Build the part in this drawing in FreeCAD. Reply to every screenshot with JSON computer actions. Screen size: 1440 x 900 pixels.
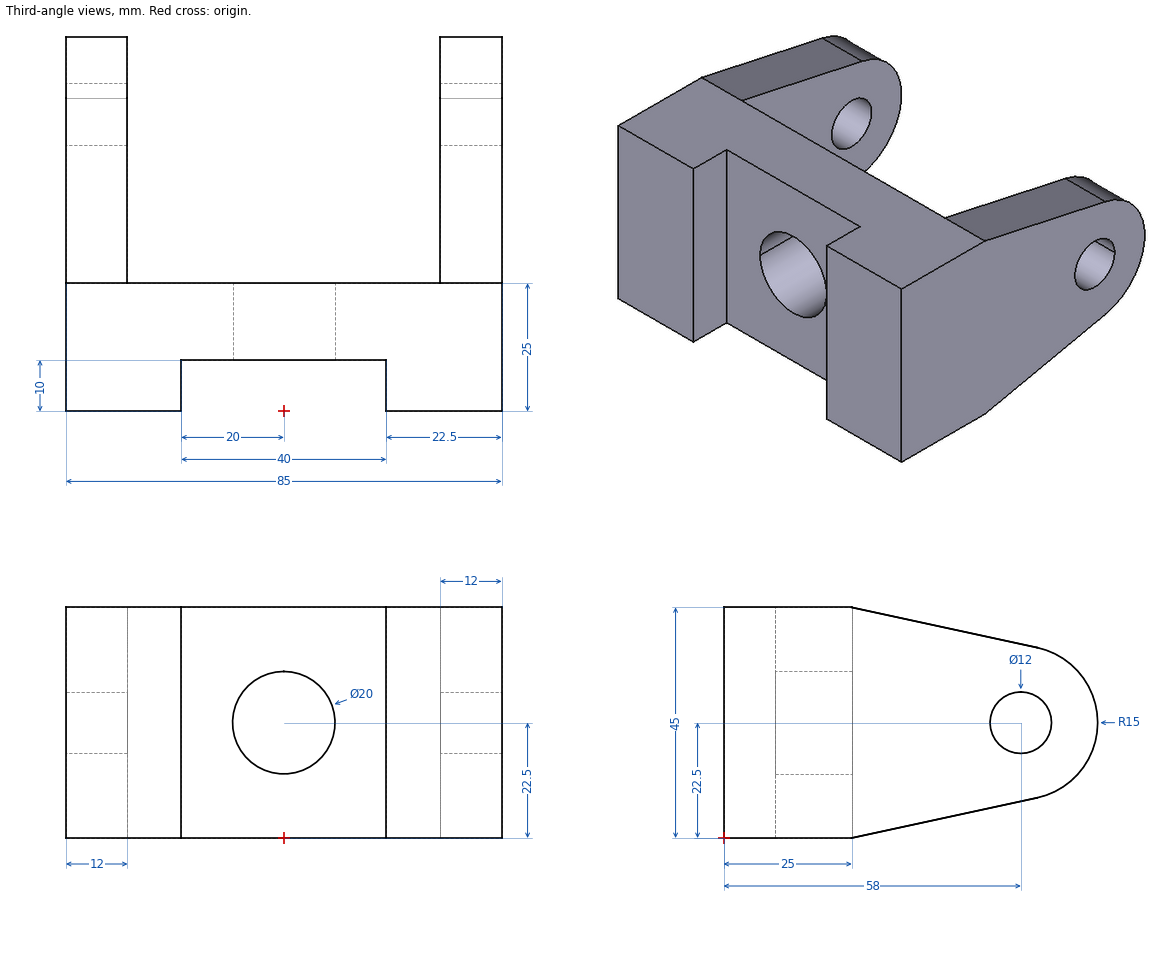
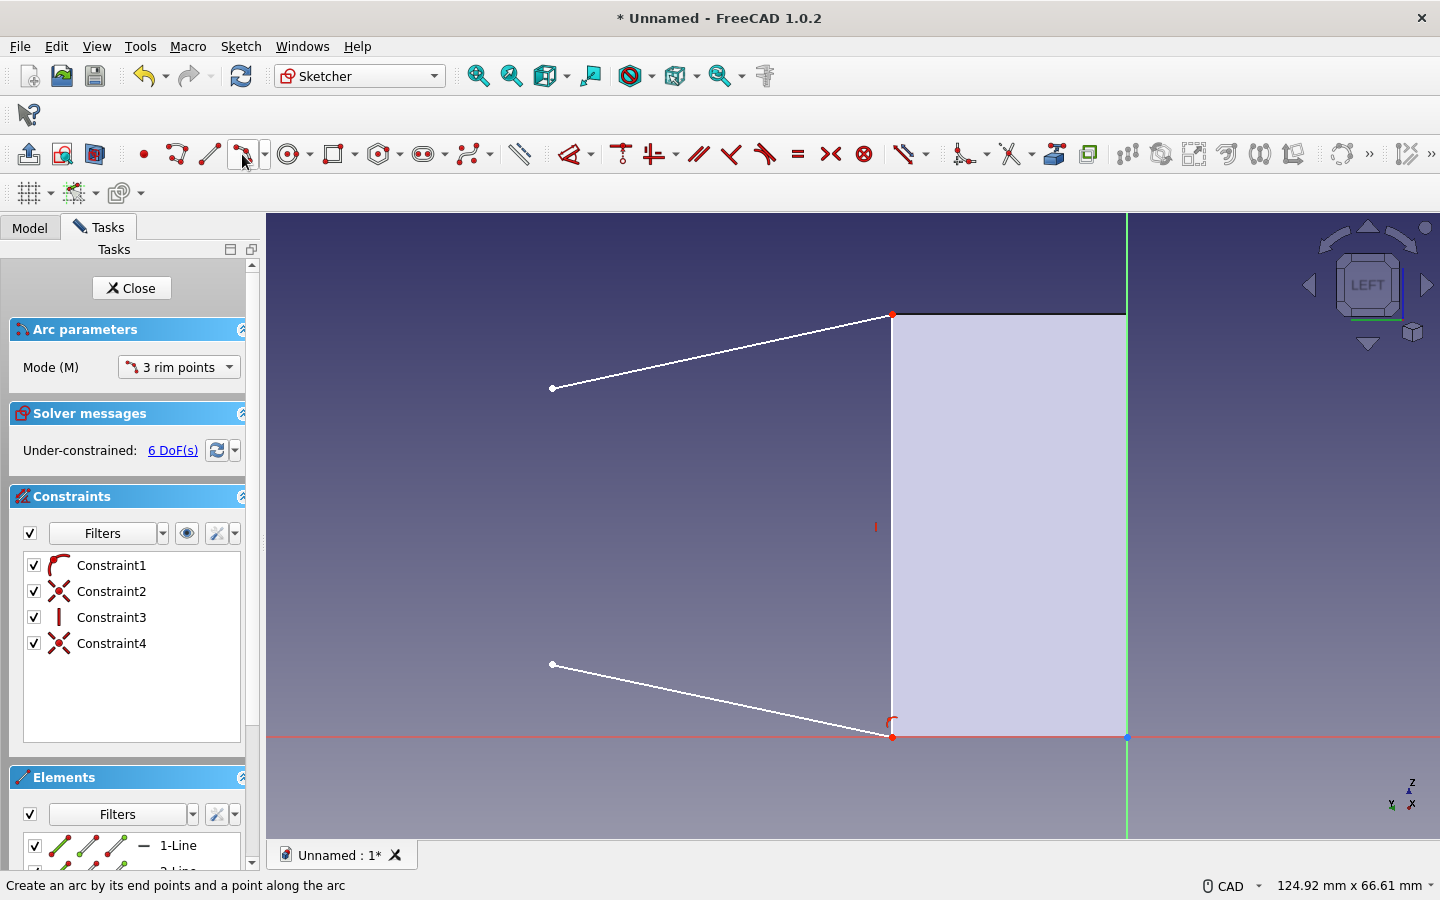
{"action": "left_click", "coordinate": [552, 389]}
{"action": "left_click", "coordinate": [552, 665]}
{"action": "left_click", "coordinate": [441, 526]}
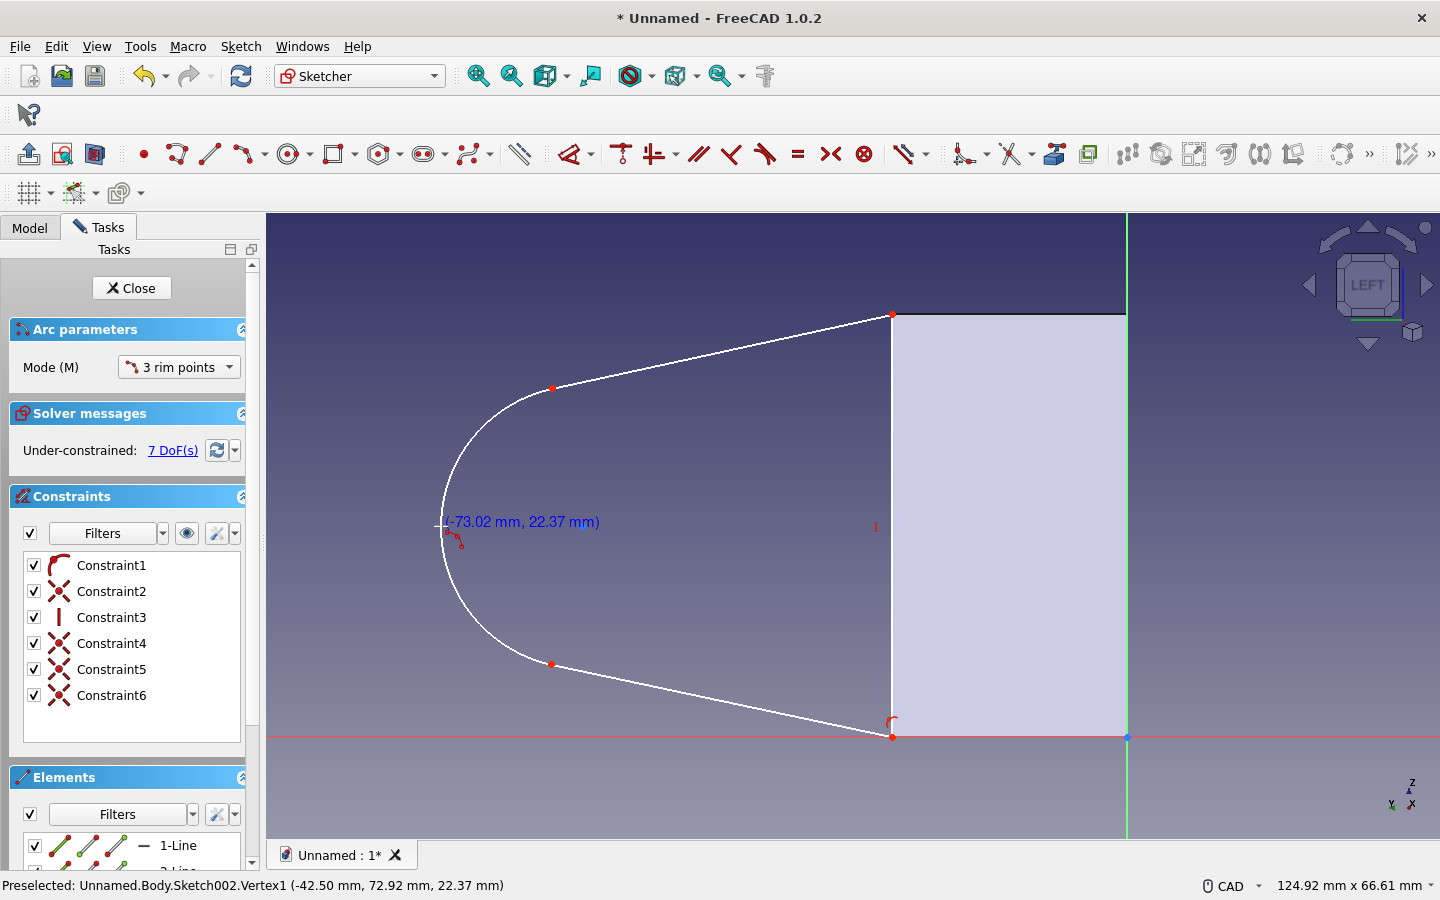
{"action": "left_click", "coordinate": [288, 154]}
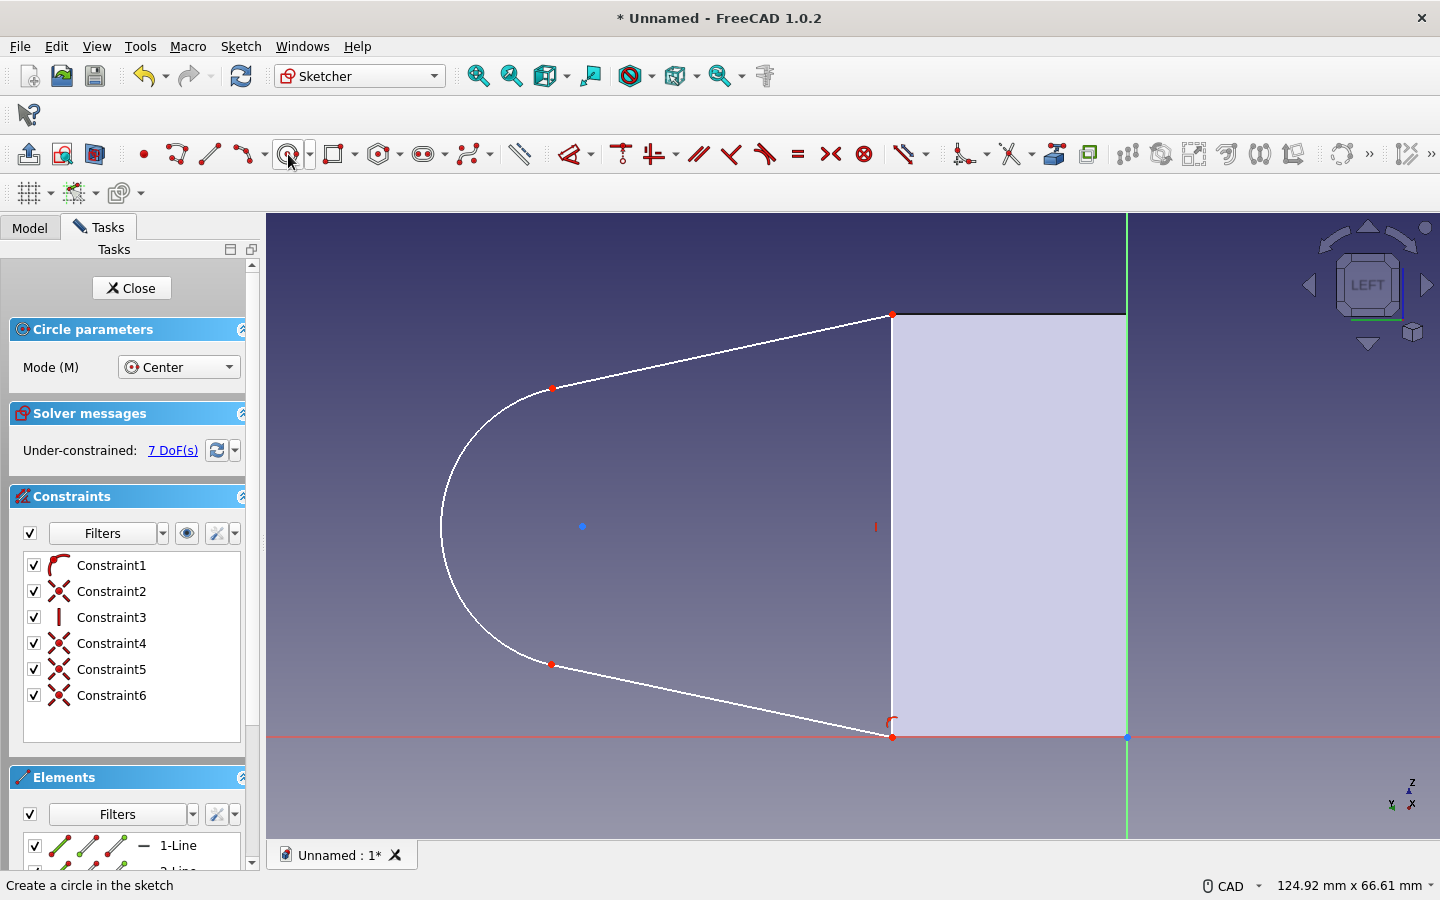
{"action": "left_click", "coordinate": [582, 526]}
{"action": "mouse_move", "coordinate": [622, 486]}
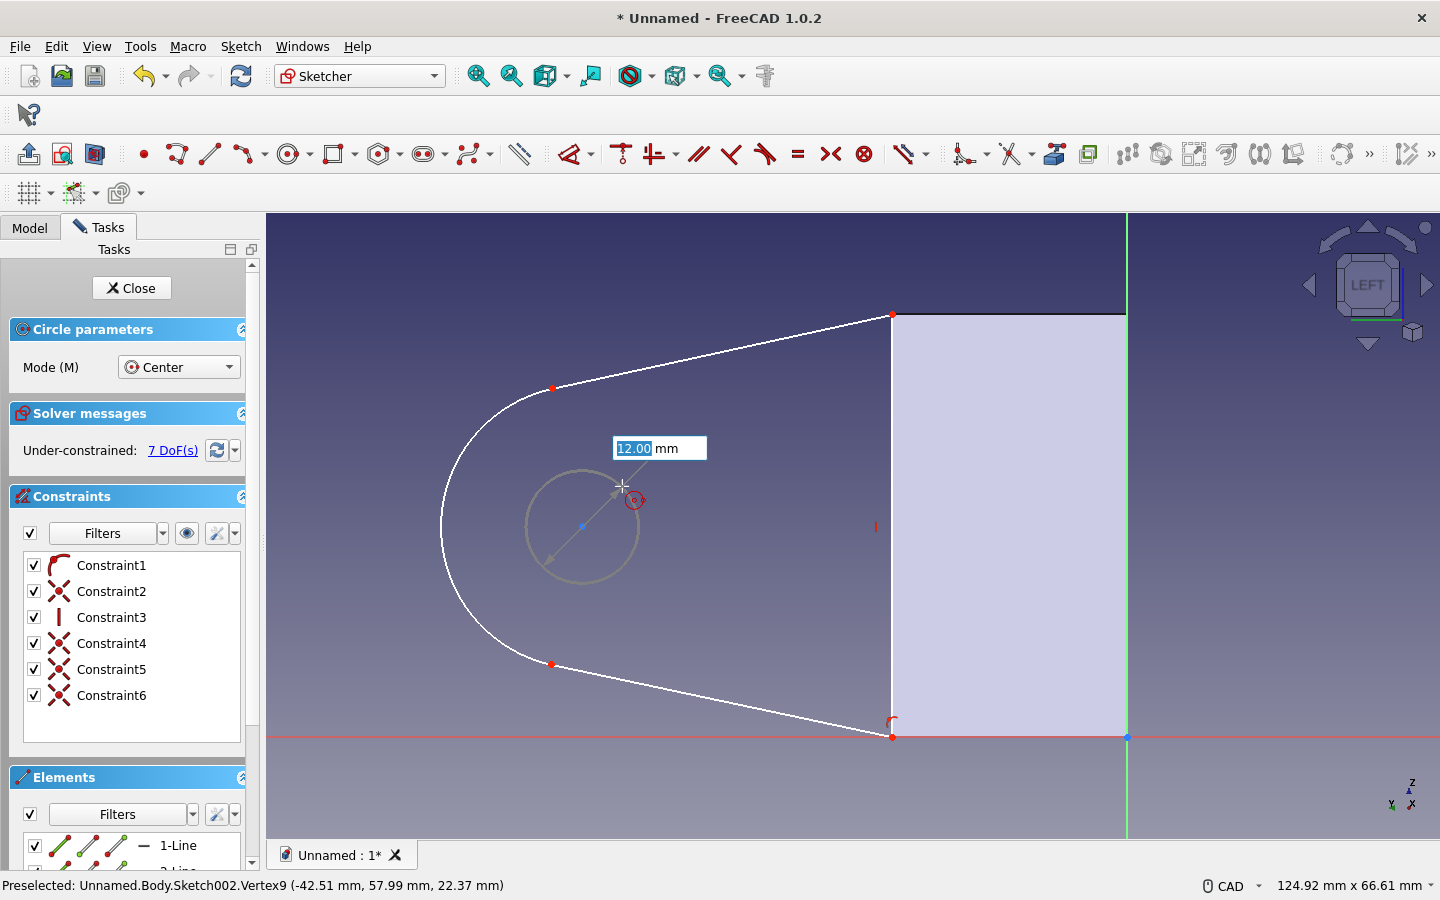
{"action": "type", "text": "12"}
{"action": "key", "text": "Return"}
{"action": "key", "text": "Escape"}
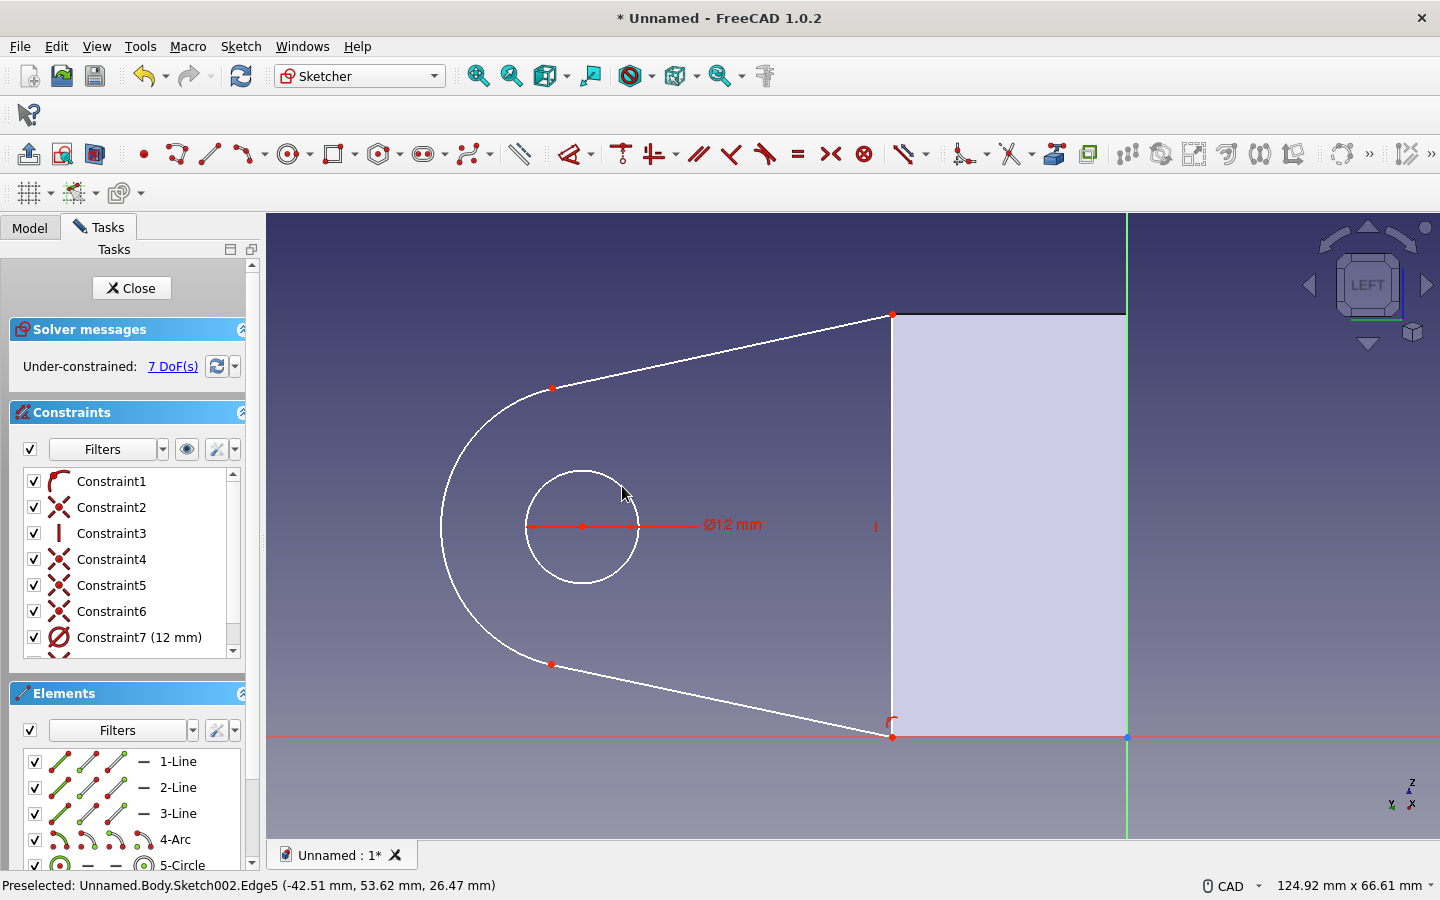
{"action": "left_click", "coordinate": [654, 687]}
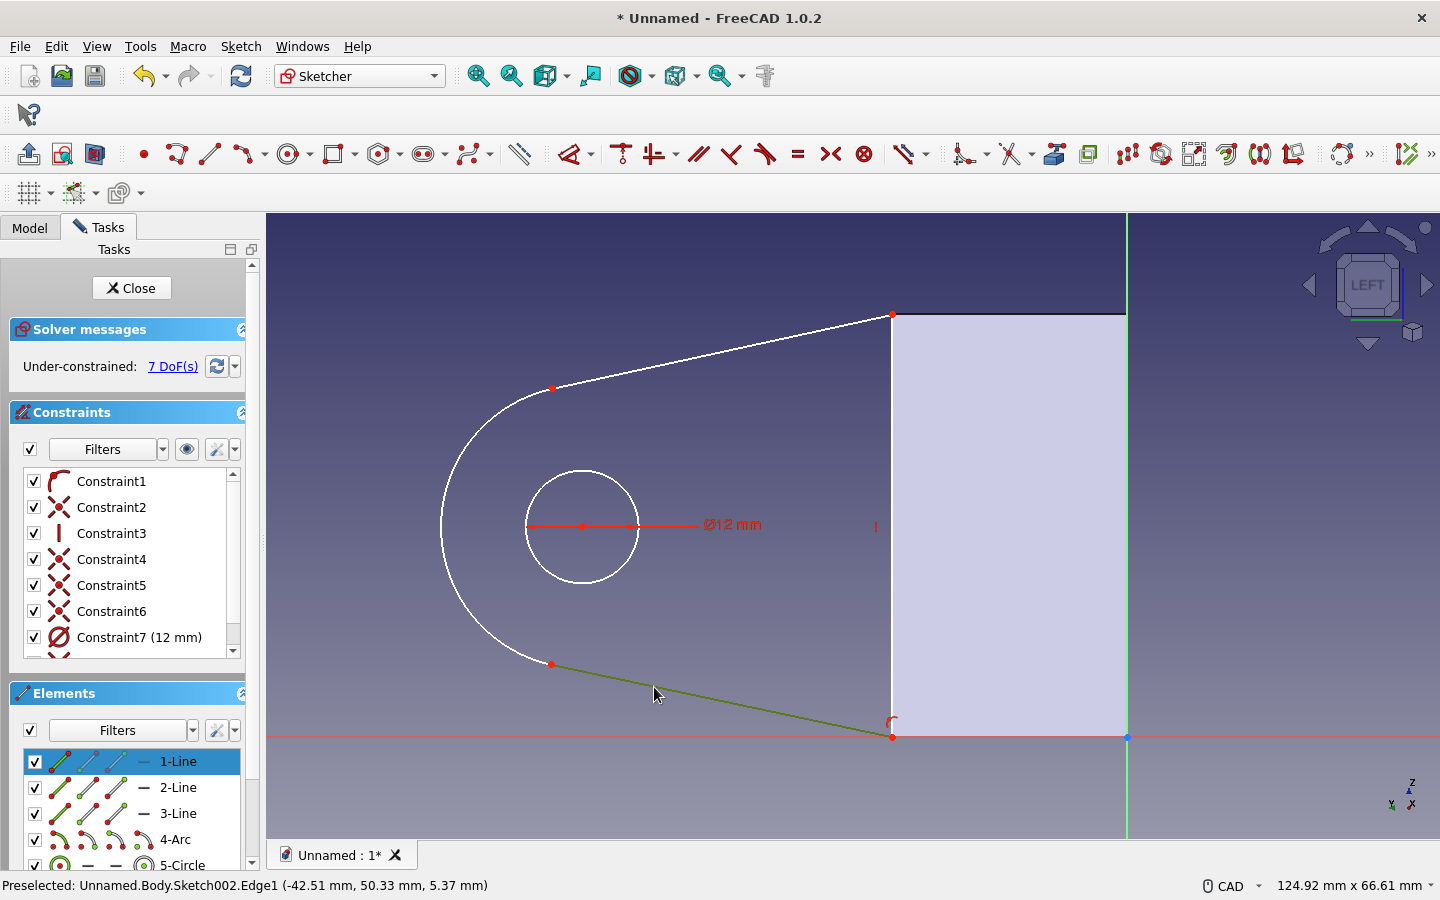
{"action": "left_click", "coordinate": [461, 454]}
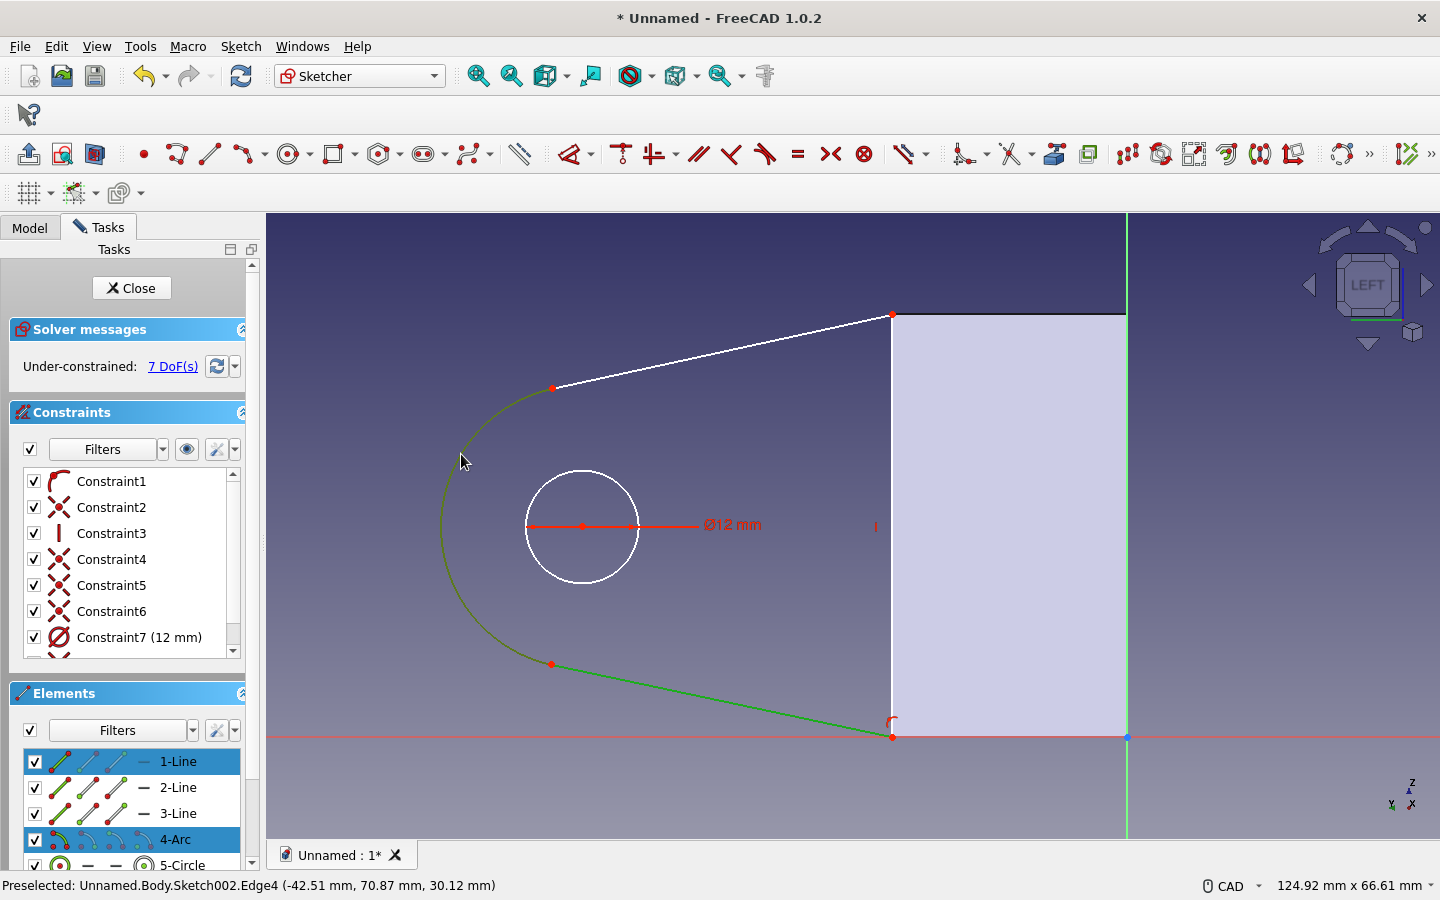
{"action": "left_click", "coordinate": [765, 154]}